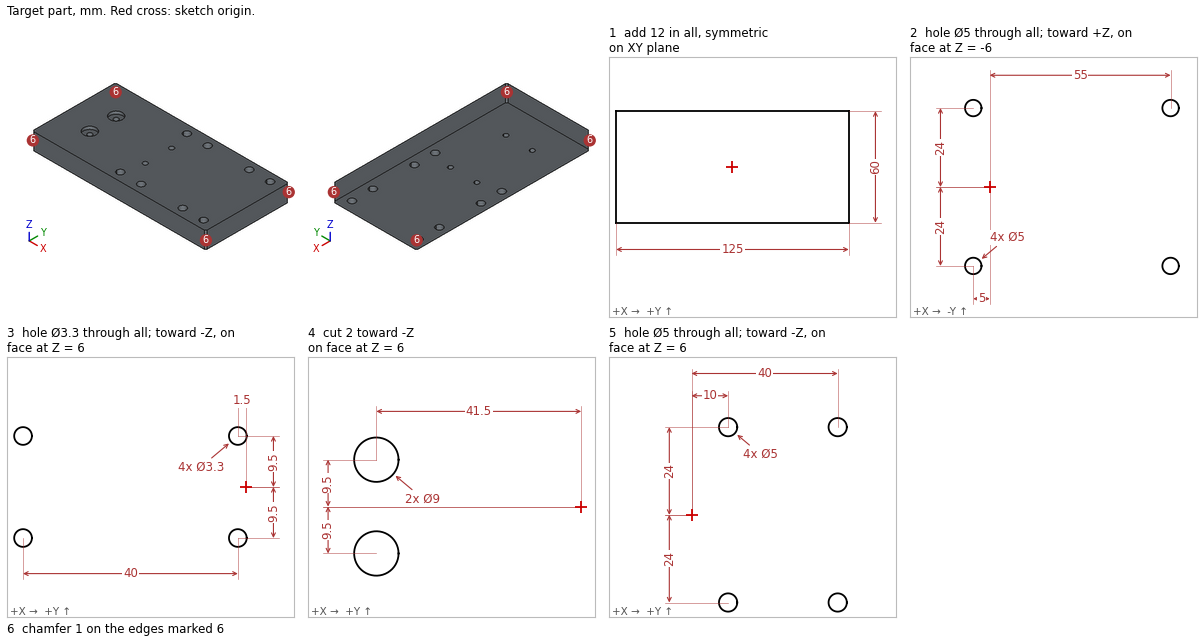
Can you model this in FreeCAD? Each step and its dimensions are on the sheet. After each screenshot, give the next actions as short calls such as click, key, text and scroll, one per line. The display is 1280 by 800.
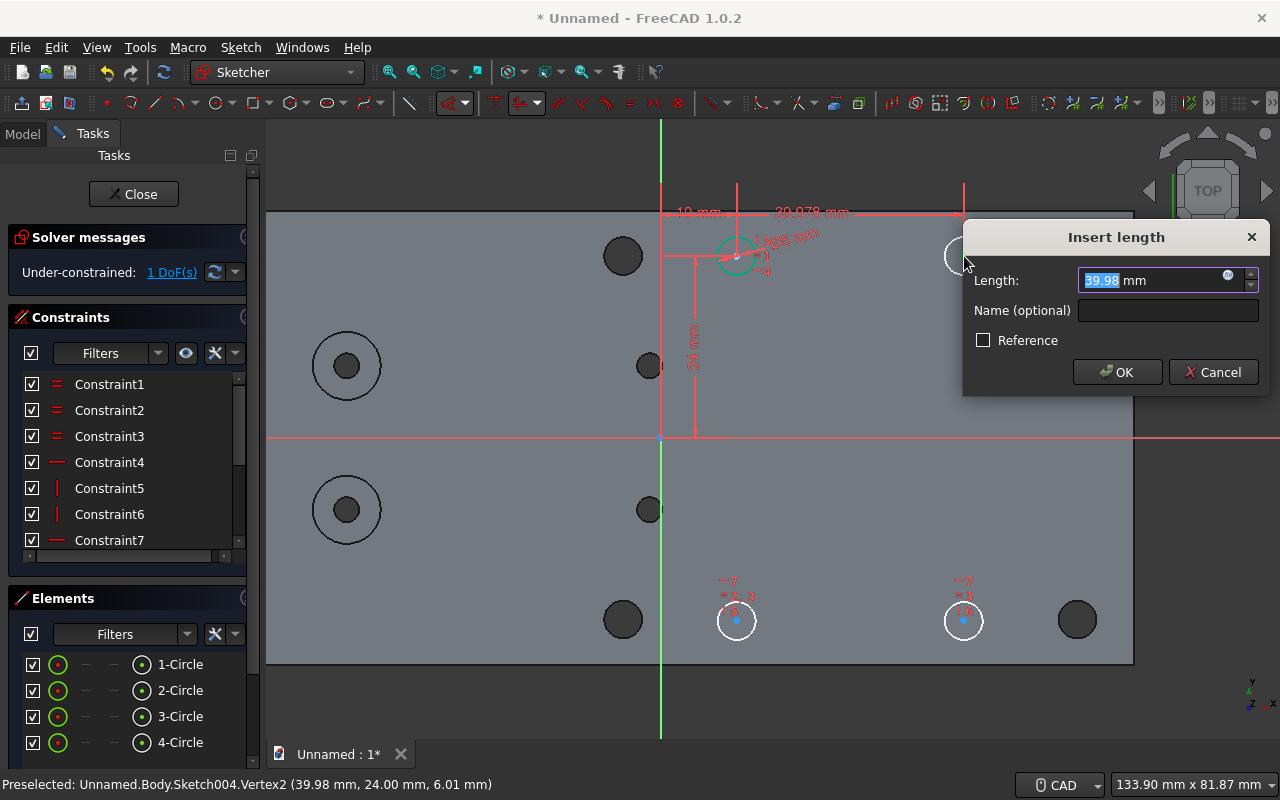
text(40)
key(Return)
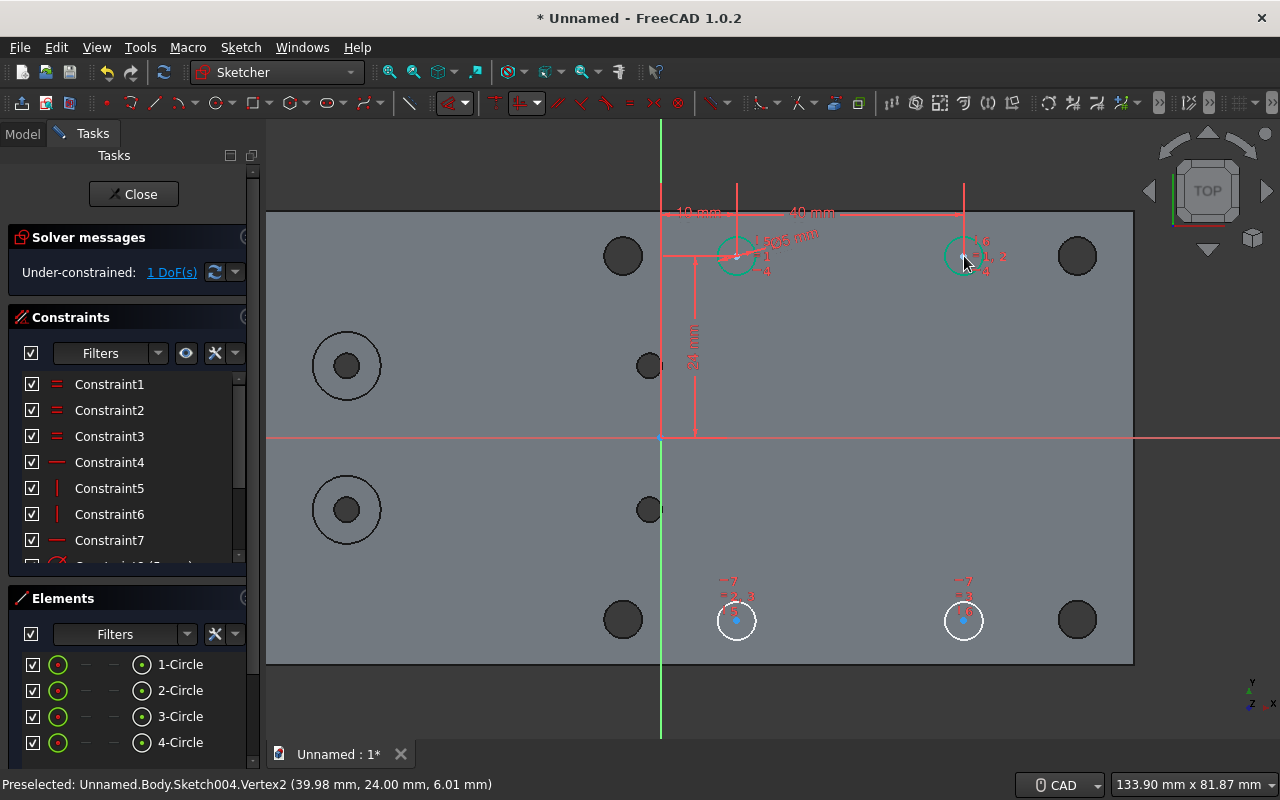
click(737, 621)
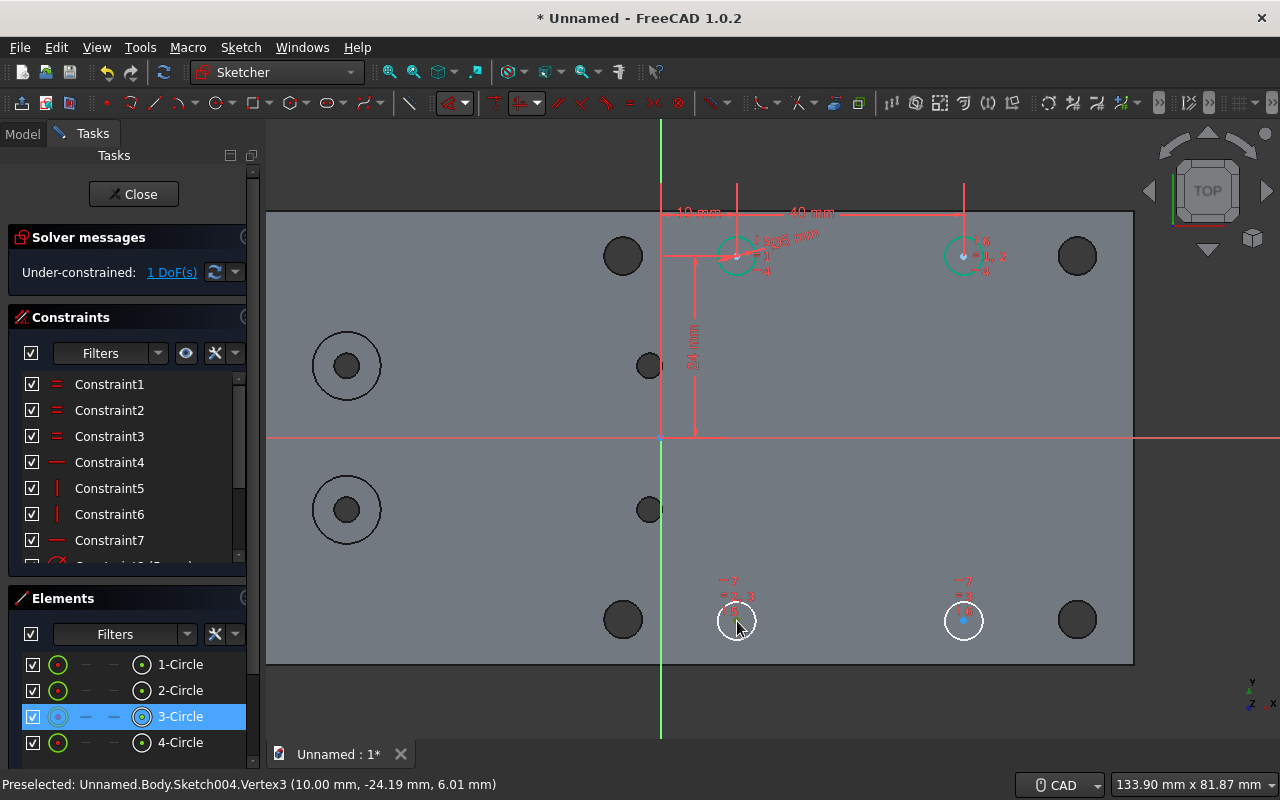
click(468, 104)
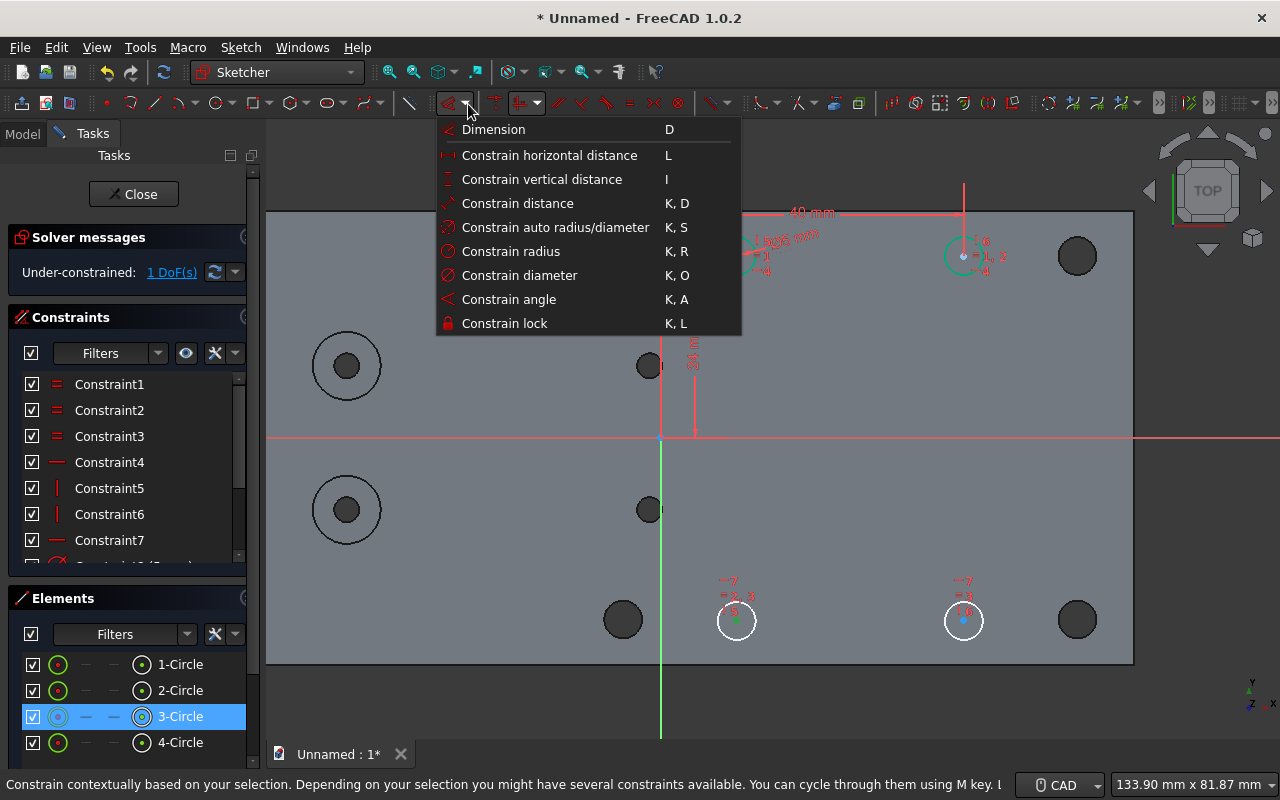
click(589, 179)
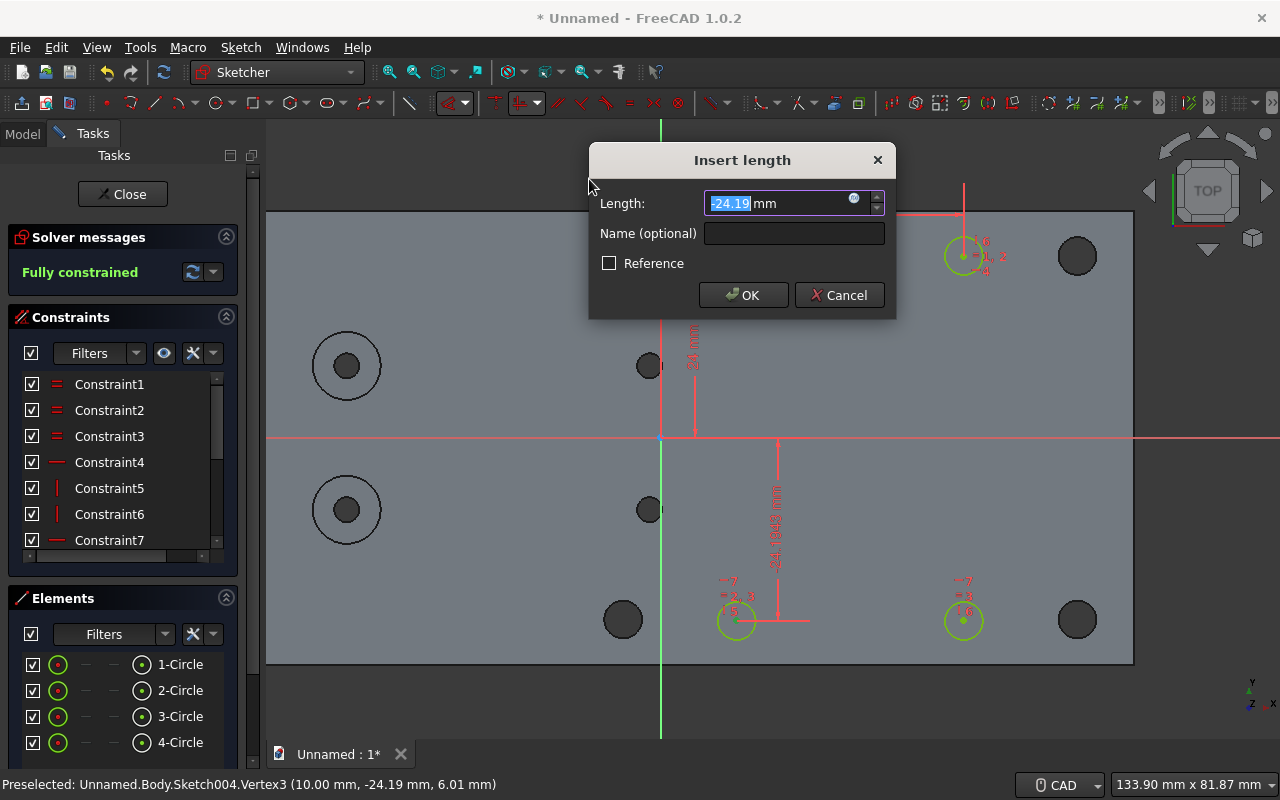
text(-24)
key(Return)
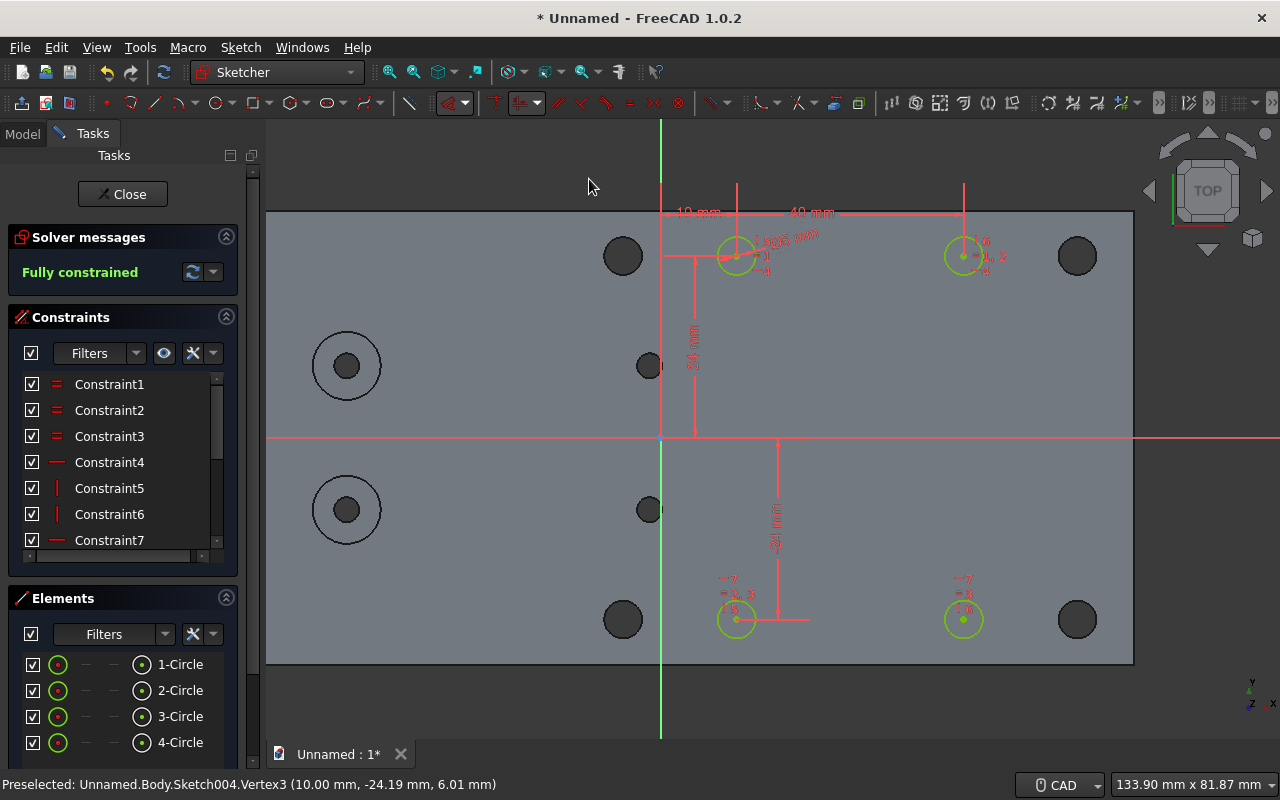
click(123, 194)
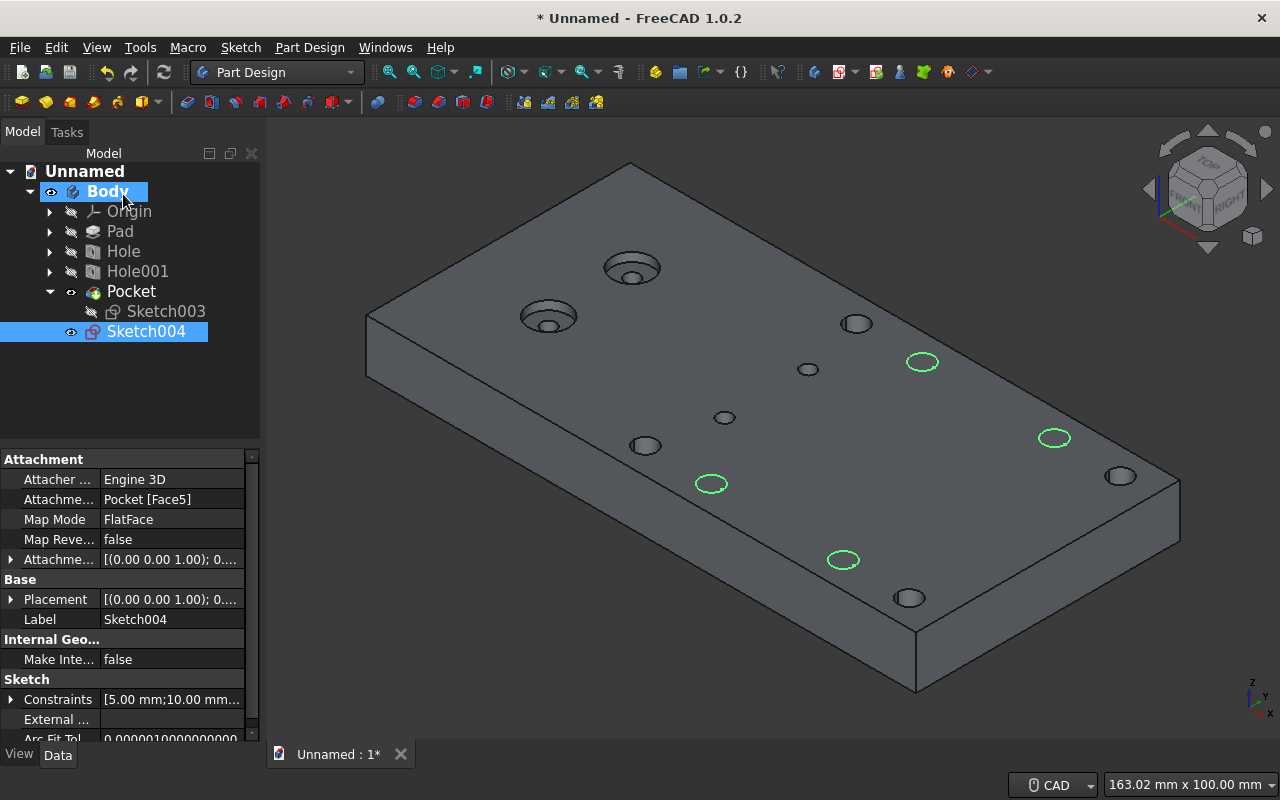
click(212, 102)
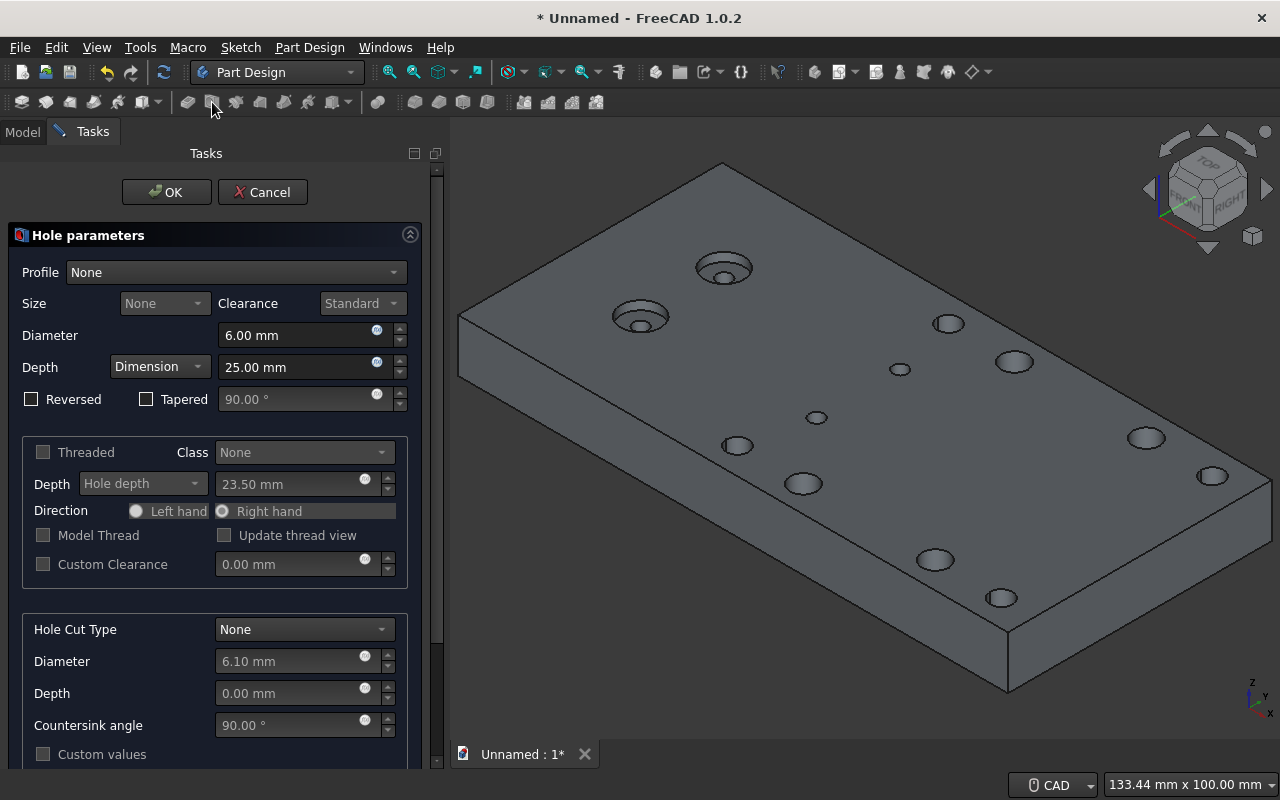
triple_click(305, 335)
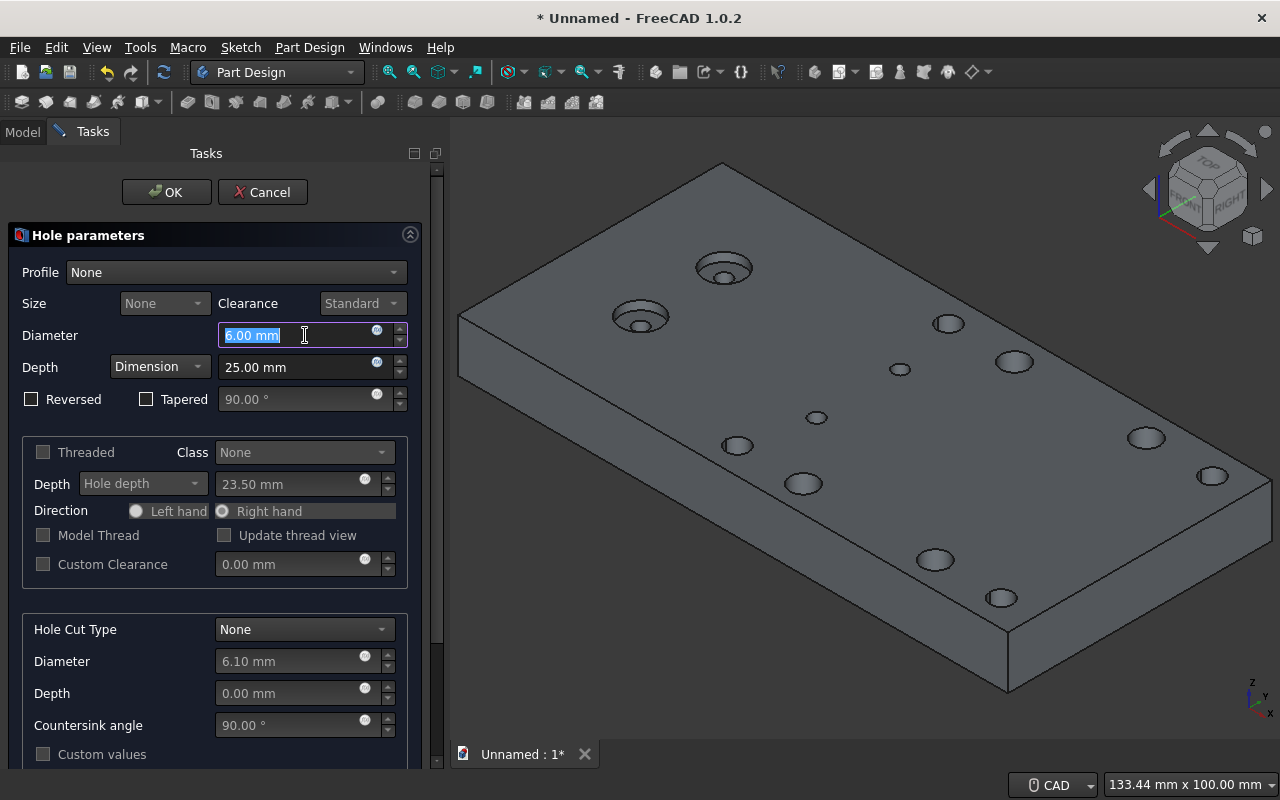
text(5)
key(Tab)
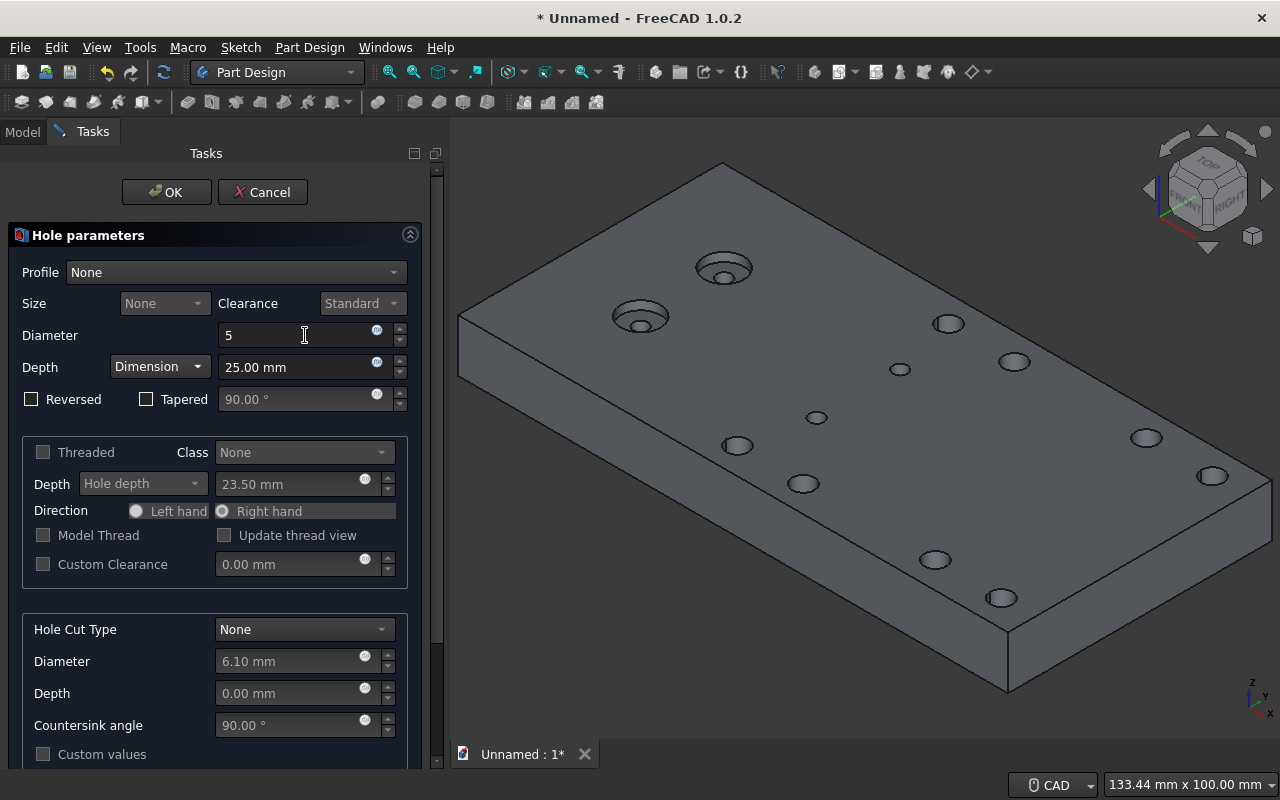
click(161, 366)